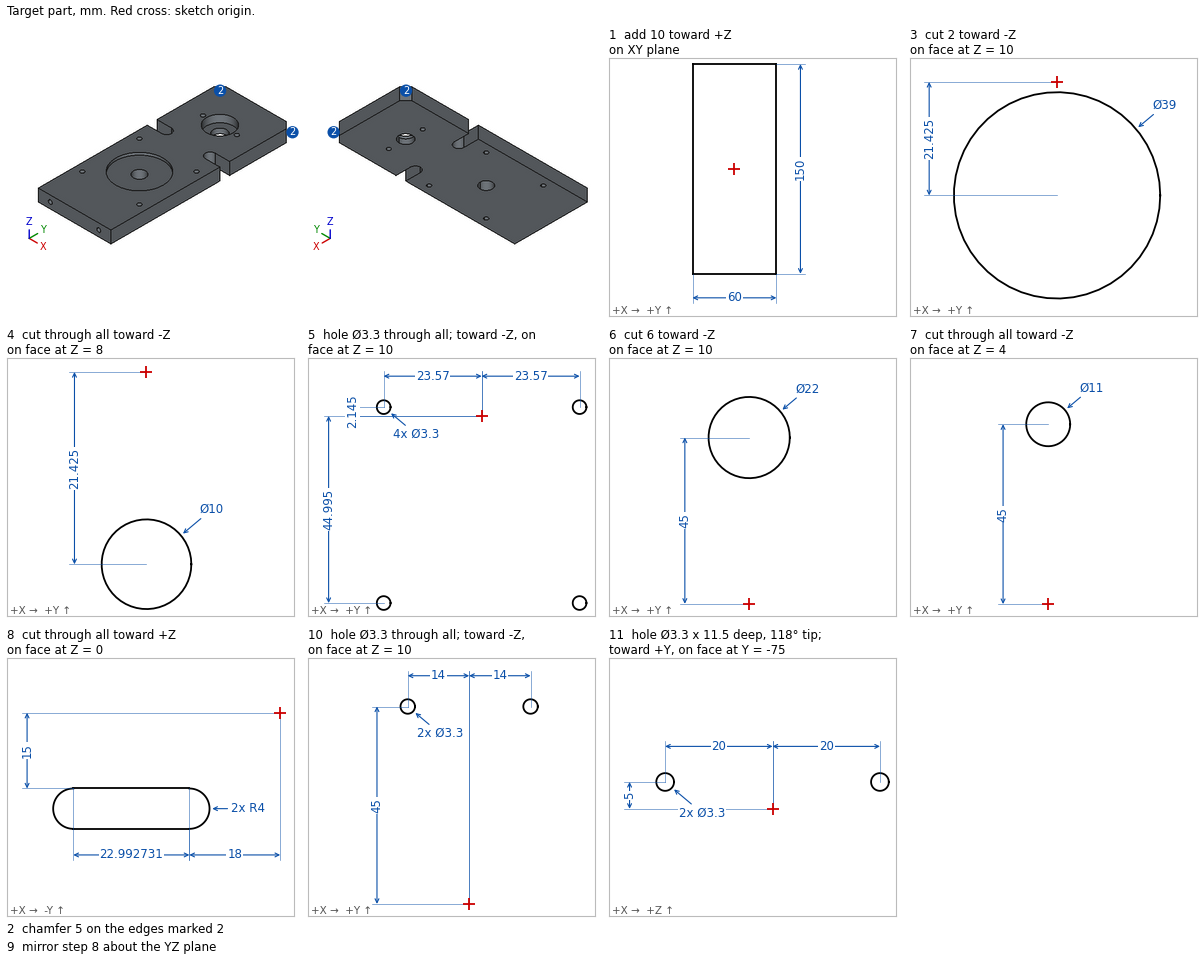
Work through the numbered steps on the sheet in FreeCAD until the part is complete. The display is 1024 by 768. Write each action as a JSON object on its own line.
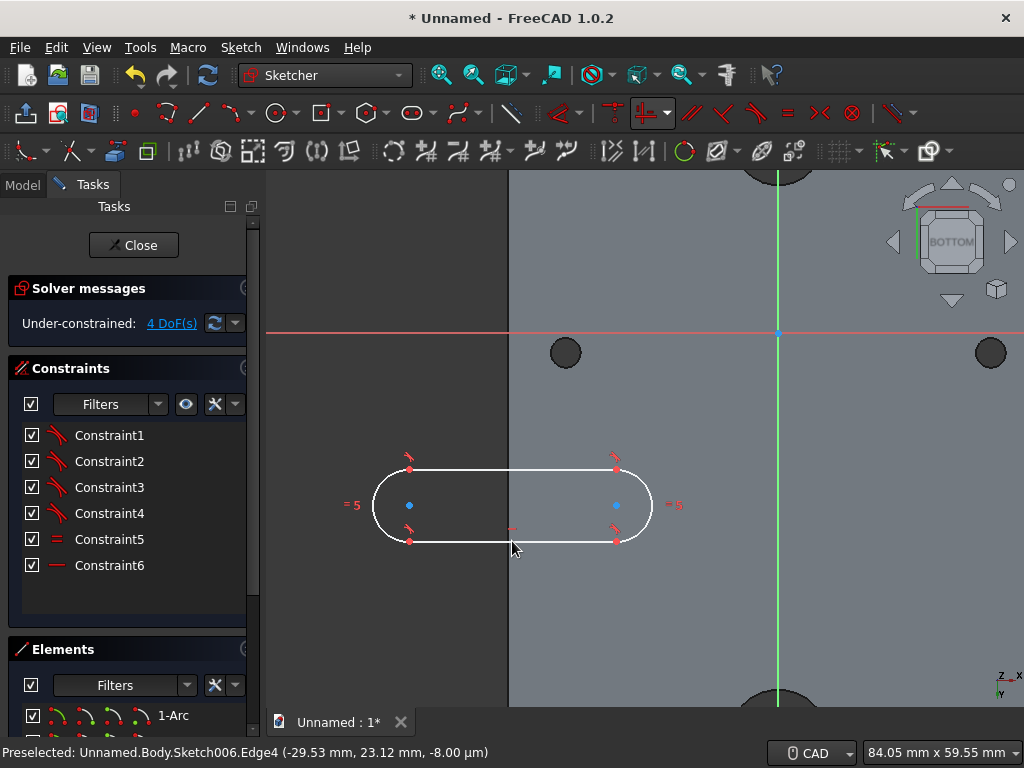
{"action": "left_click", "coordinate": [558, 114]}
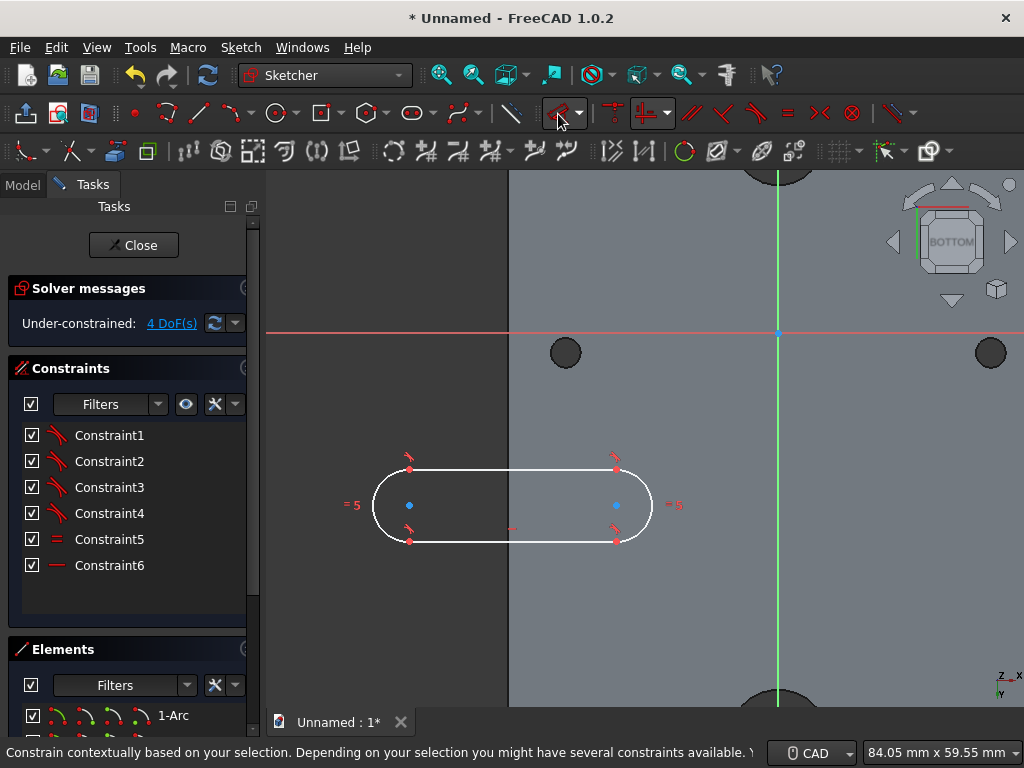
{"action": "left_click", "coordinate": [380, 485]}
{"action": "left_click", "coordinate": [354, 466]}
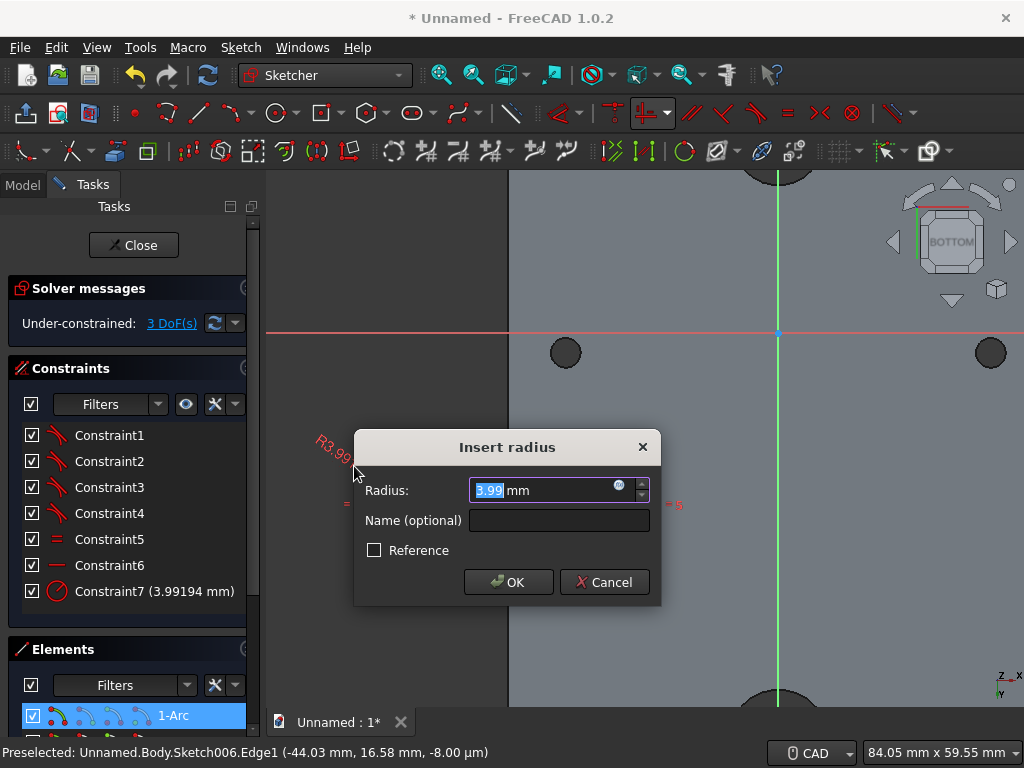
{"action": "type", "text": "4"}
{"action": "key", "text": "Return"}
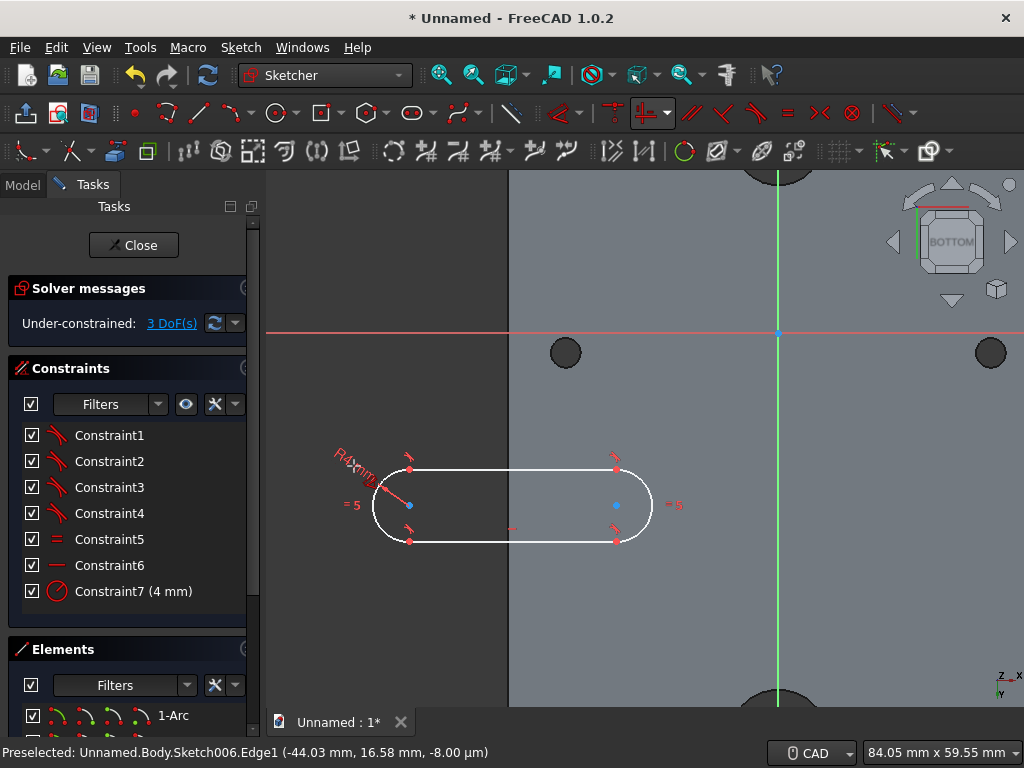
{"action": "left_click", "coordinate": [409, 470]}
{"action": "left_click", "coordinate": [812, 402]}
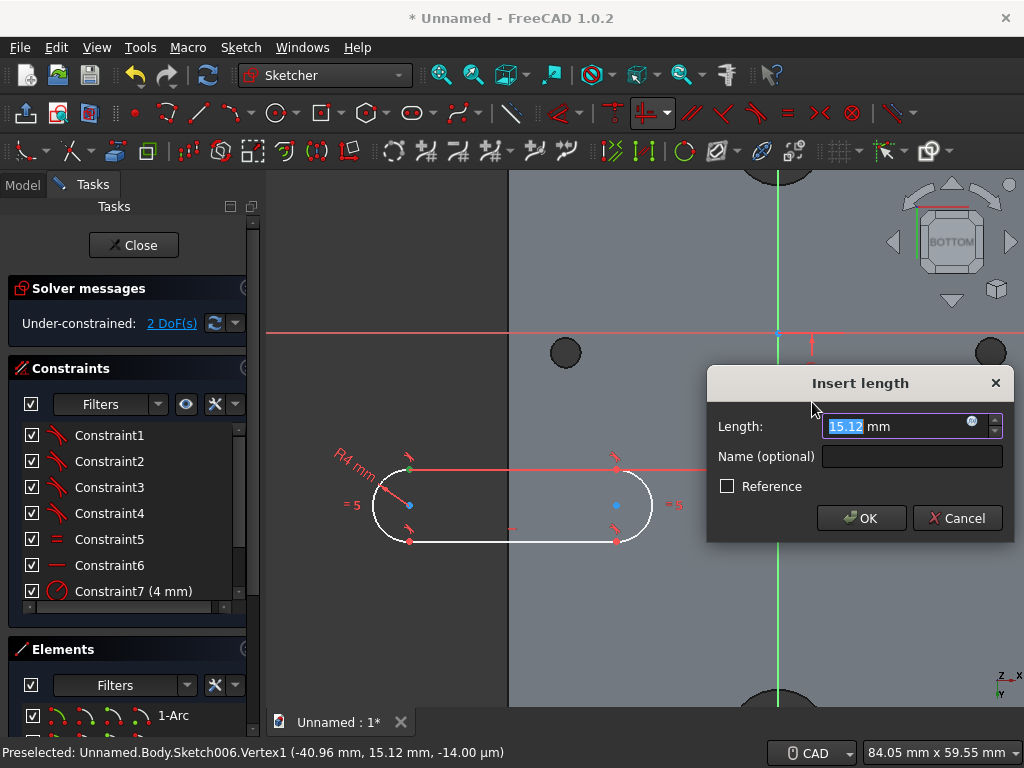
{"action": "type", "text": "15"}
{"action": "key", "text": "Return"}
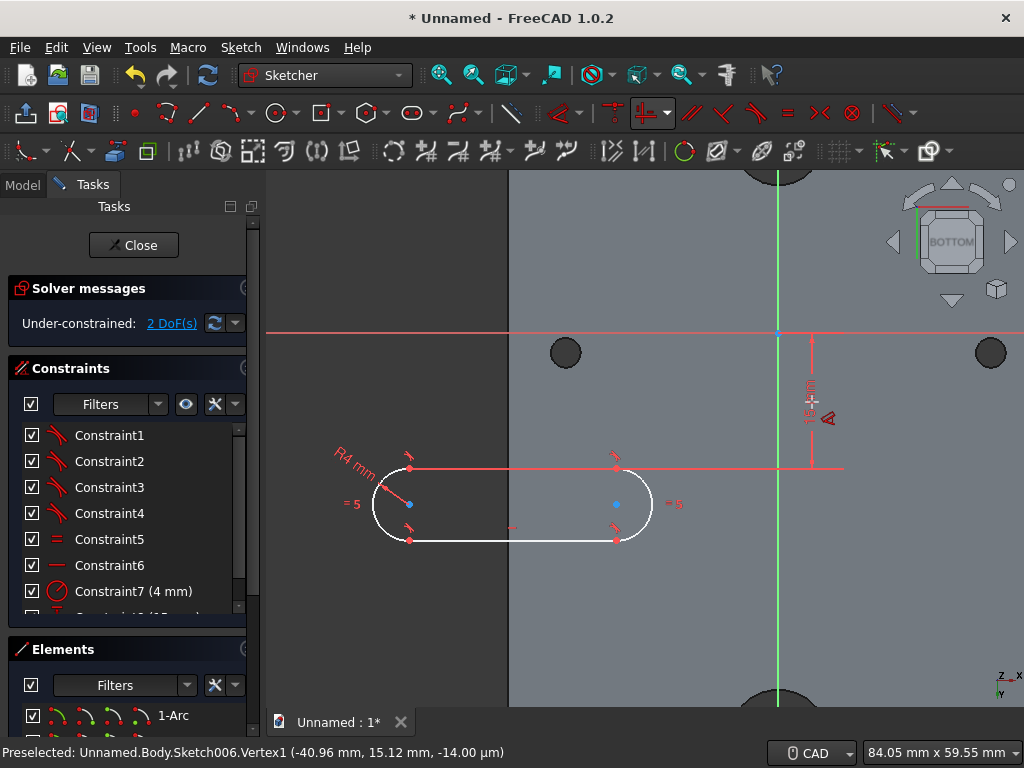
{"action": "left_click", "coordinate": [616, 541]}
{"action": "left_click", "coordinate": [697, 575]}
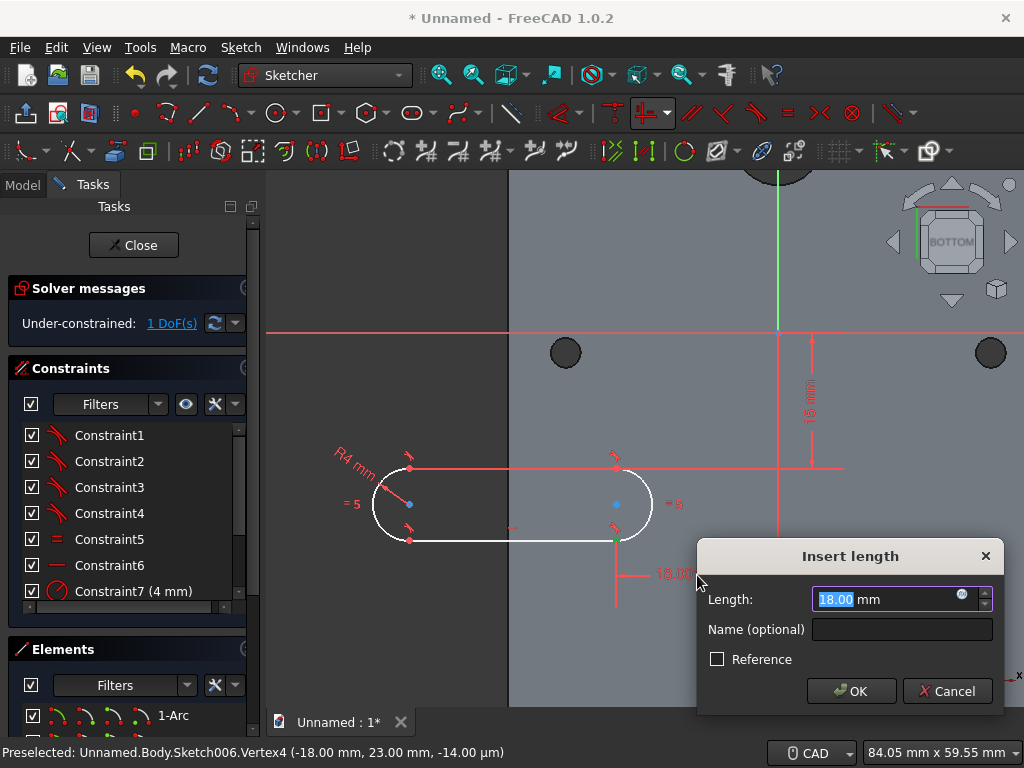
{"action": "type", "text": "18"}
{"action": "key", "text": "Return"}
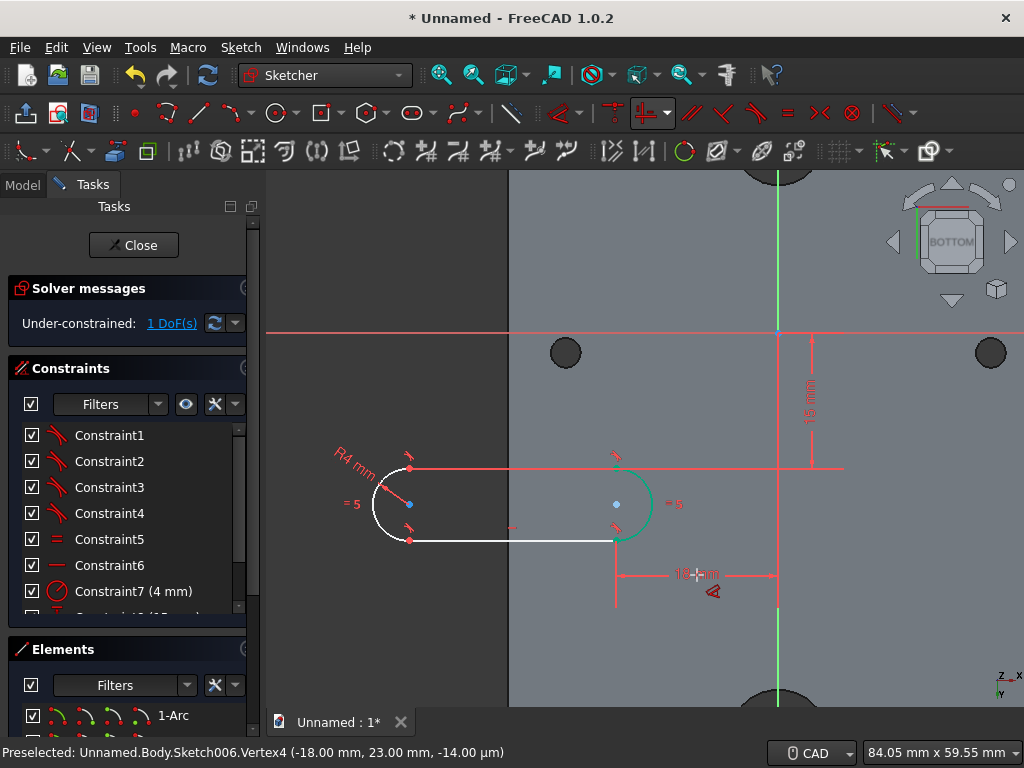
{"action": "left_click", "coordinate": [471, 469]}
{"action": "left_click", "coordinate": [513, 503]}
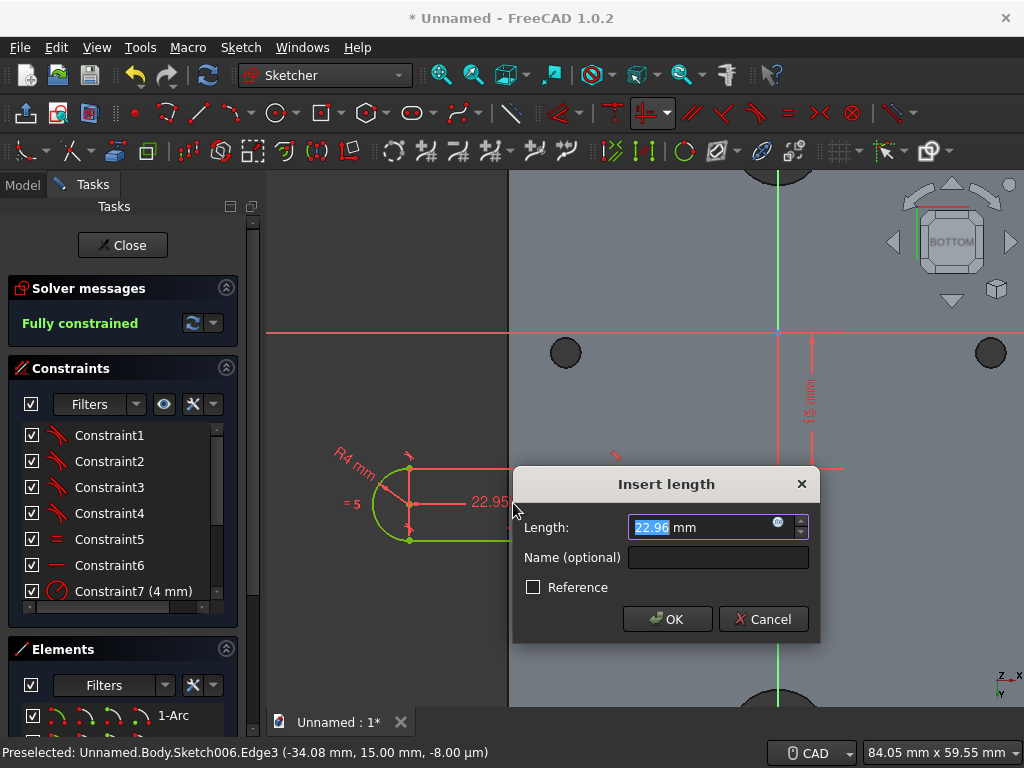
{"action": "type", "text": "22.992731"}
{"action": "key", "text": "Return"}
{"action": "key", "text": "Escape"}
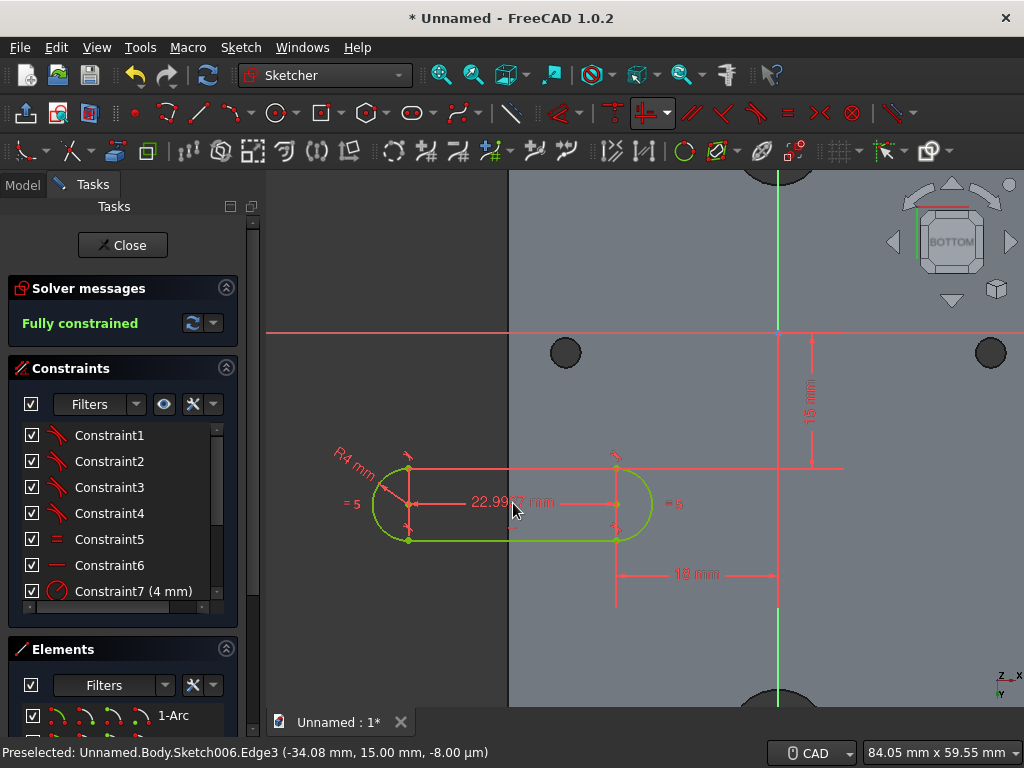
{"action": "left_click", "coordinate": [123, 245]}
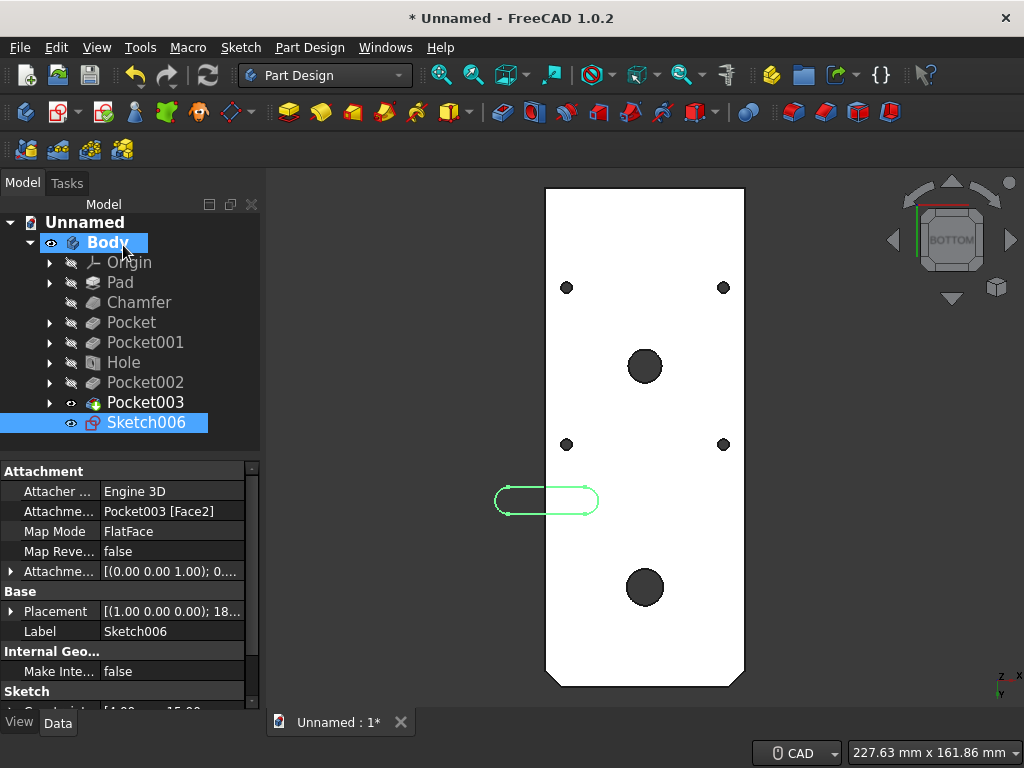
{"action": "left_click", "coordinate": [504, 112]}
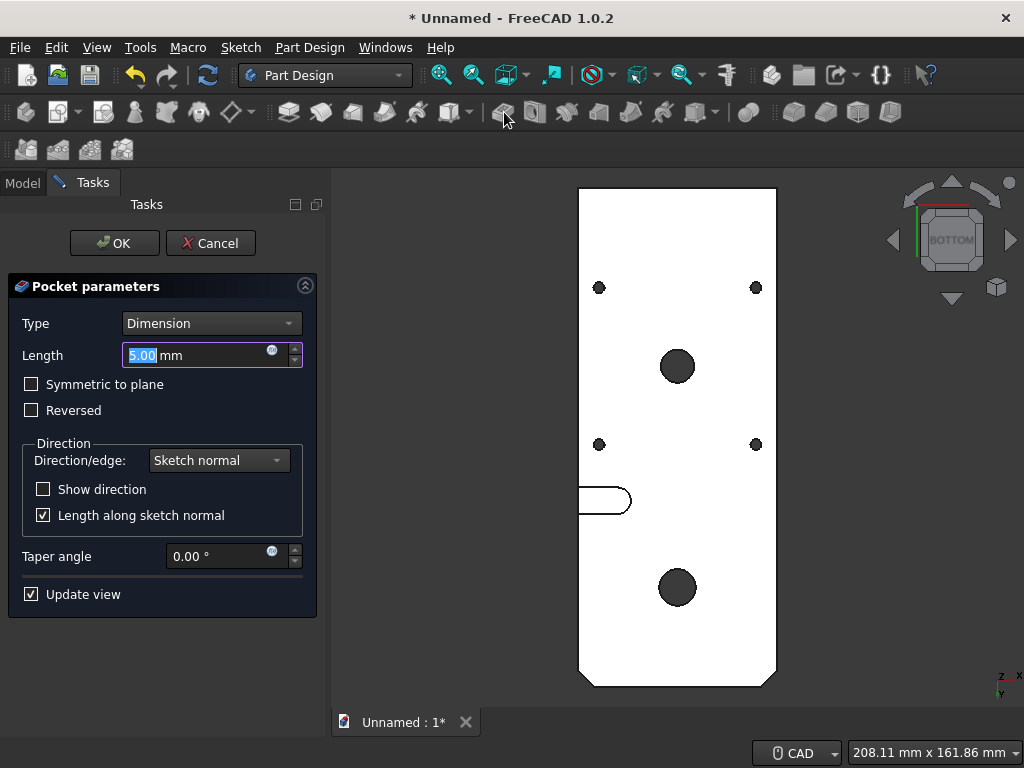
{"action": "left_click", "coordinate": [212, 324]}